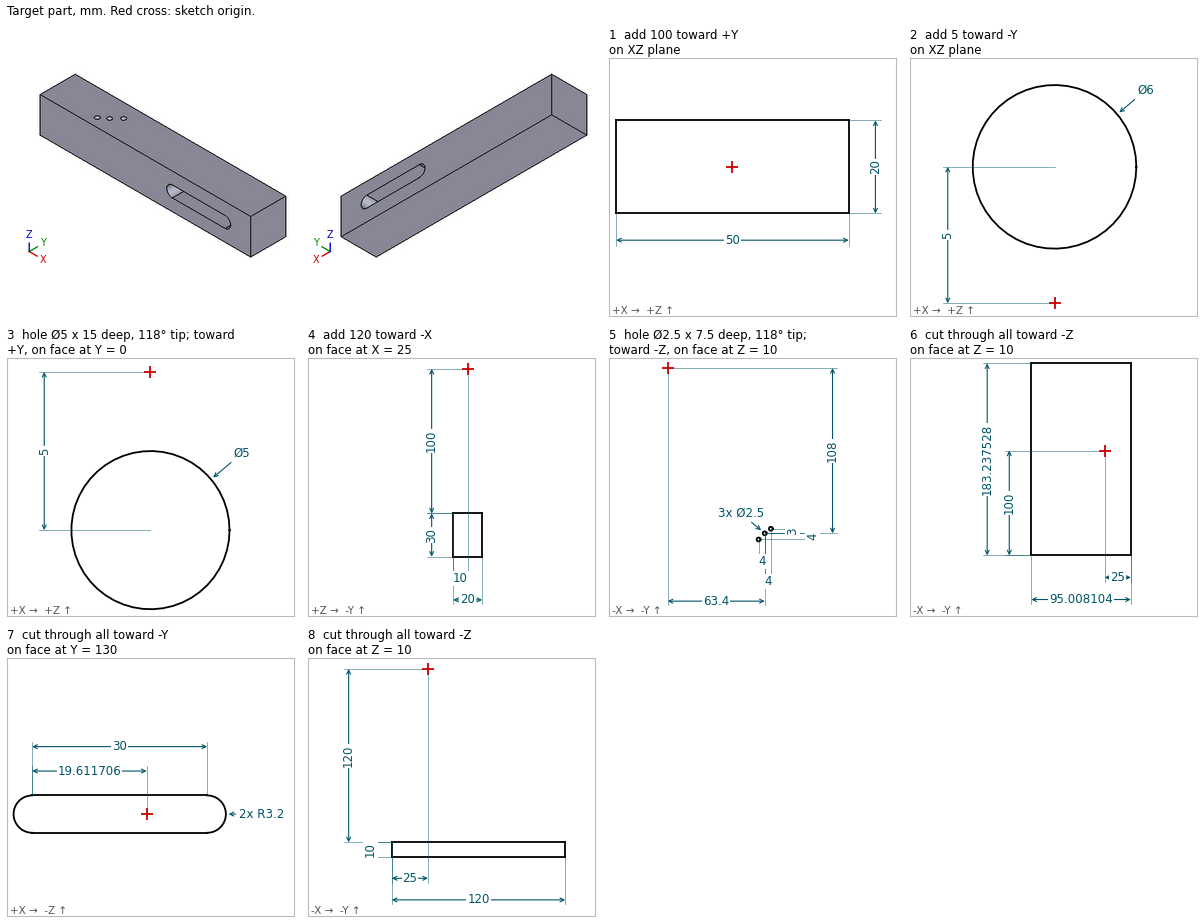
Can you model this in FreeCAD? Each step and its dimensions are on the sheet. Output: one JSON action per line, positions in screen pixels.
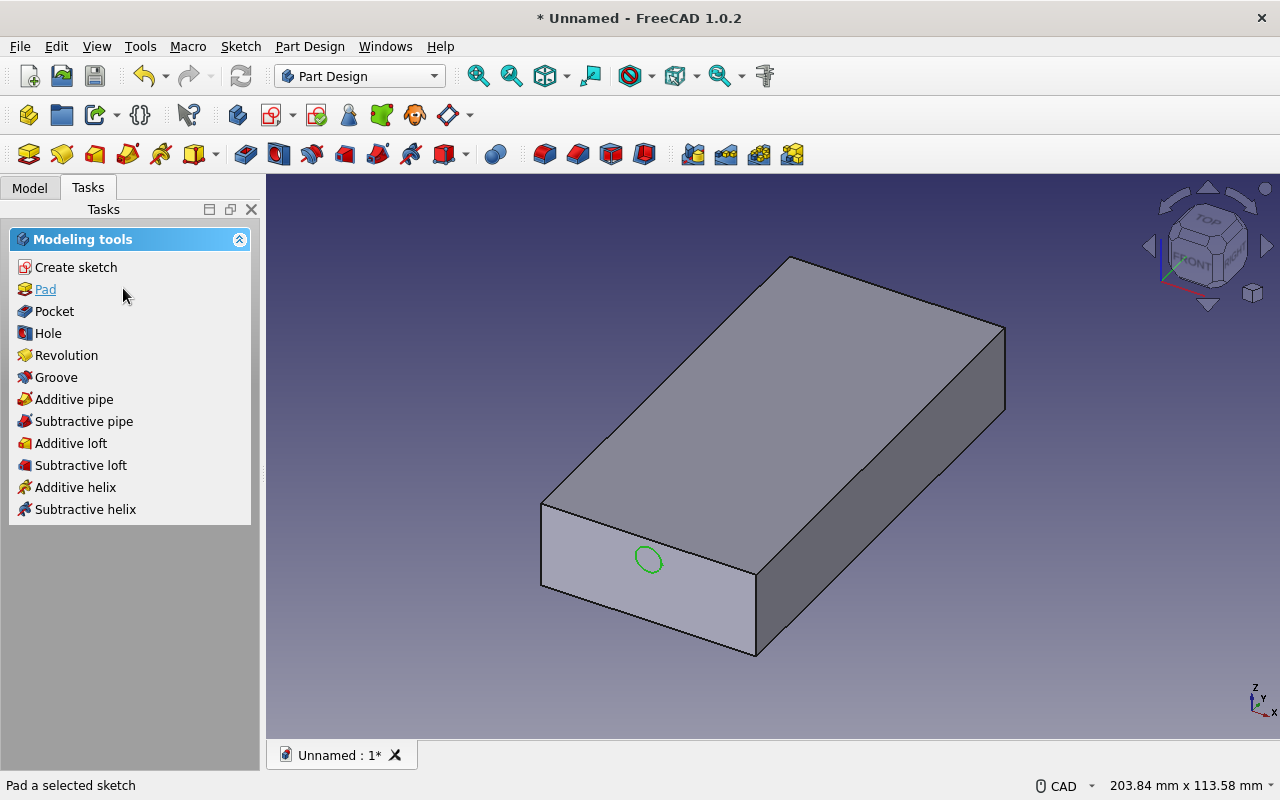
{"action": "left_click", "coordinate": [29, 154]}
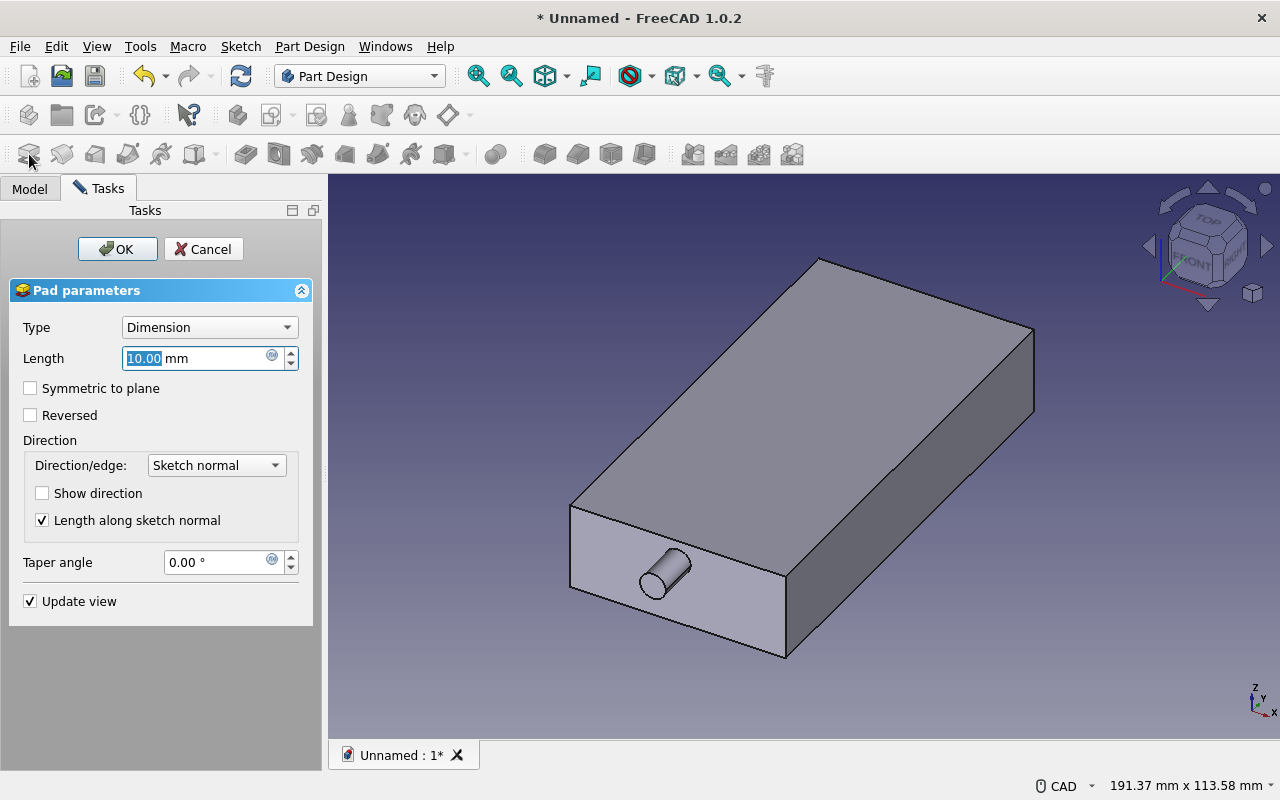
{"action": "type", "text": "5"}
{"action": "key", "text": "Tab"}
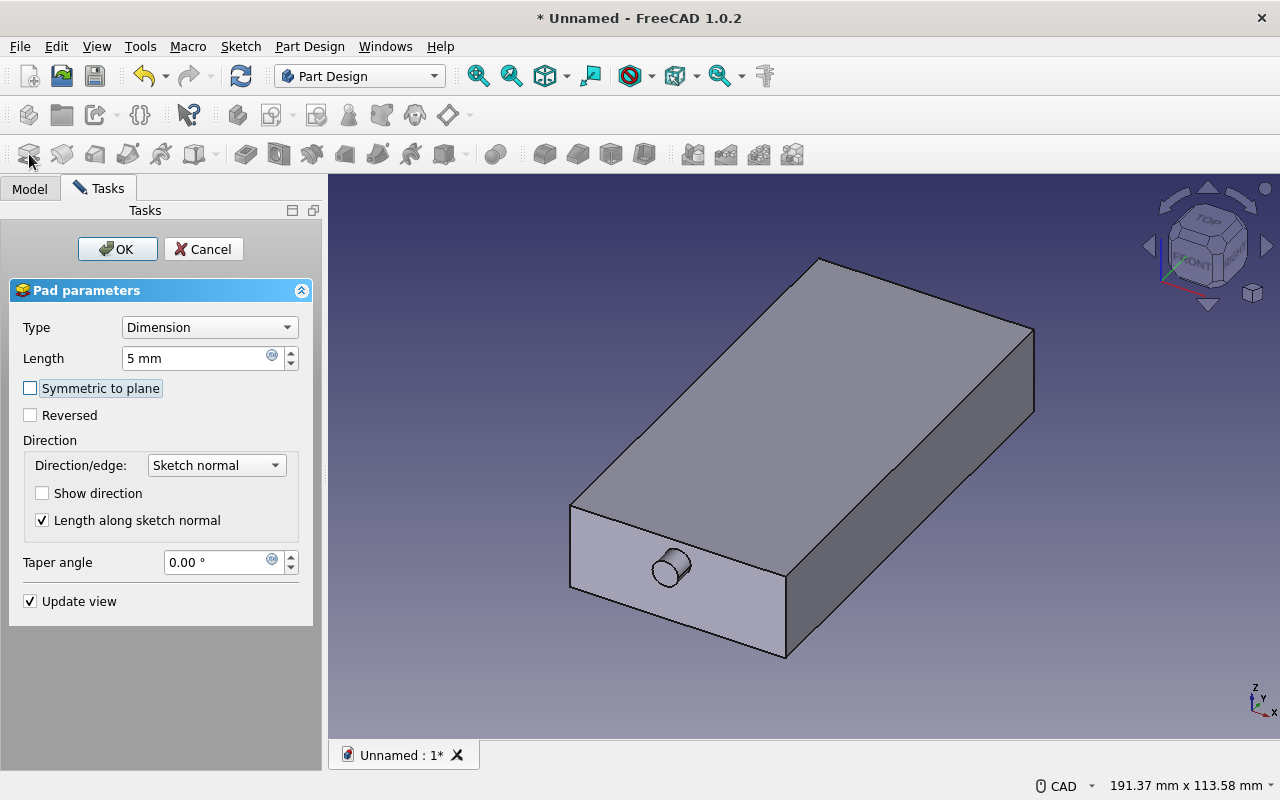
{"action": "left_click", "coordinate": [118, 249]}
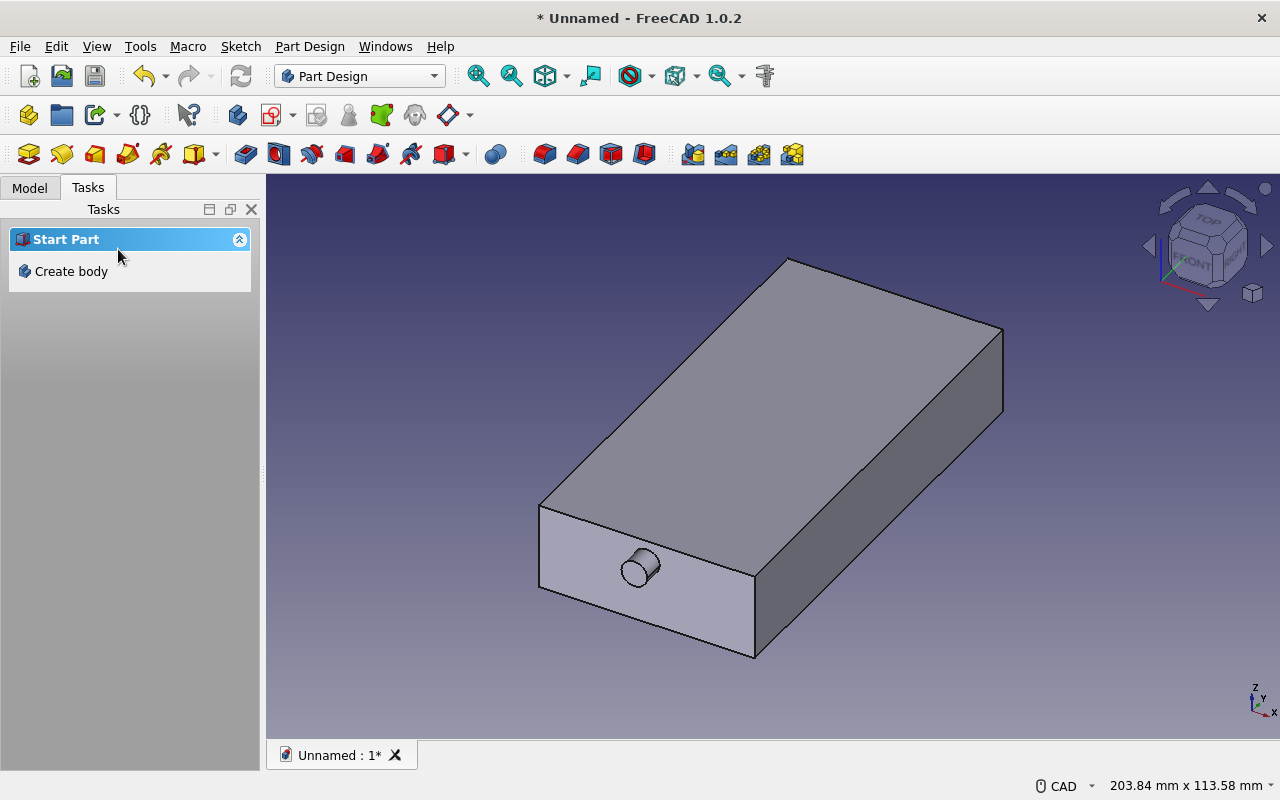
{"action": "left_click", "coordinate": [708, 601]}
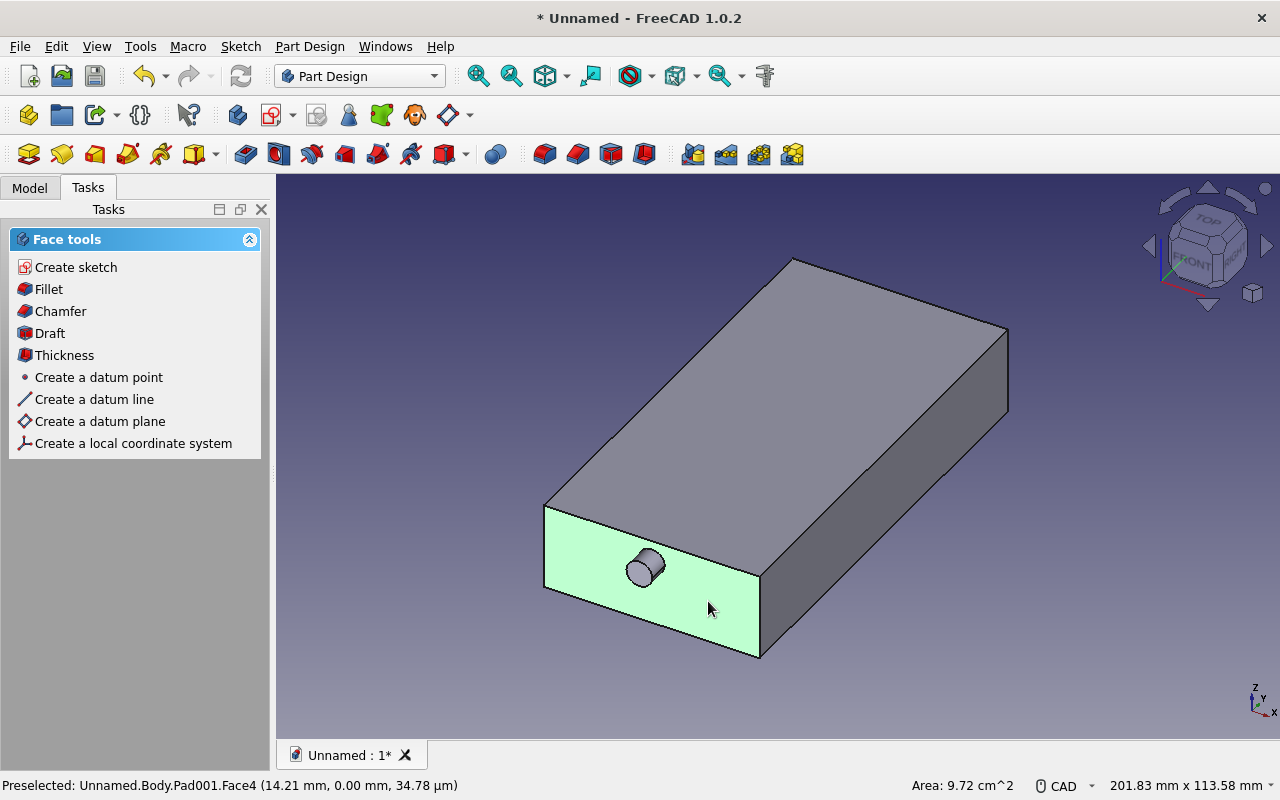
{"action": "left_click", "coordinate": [270, 116]}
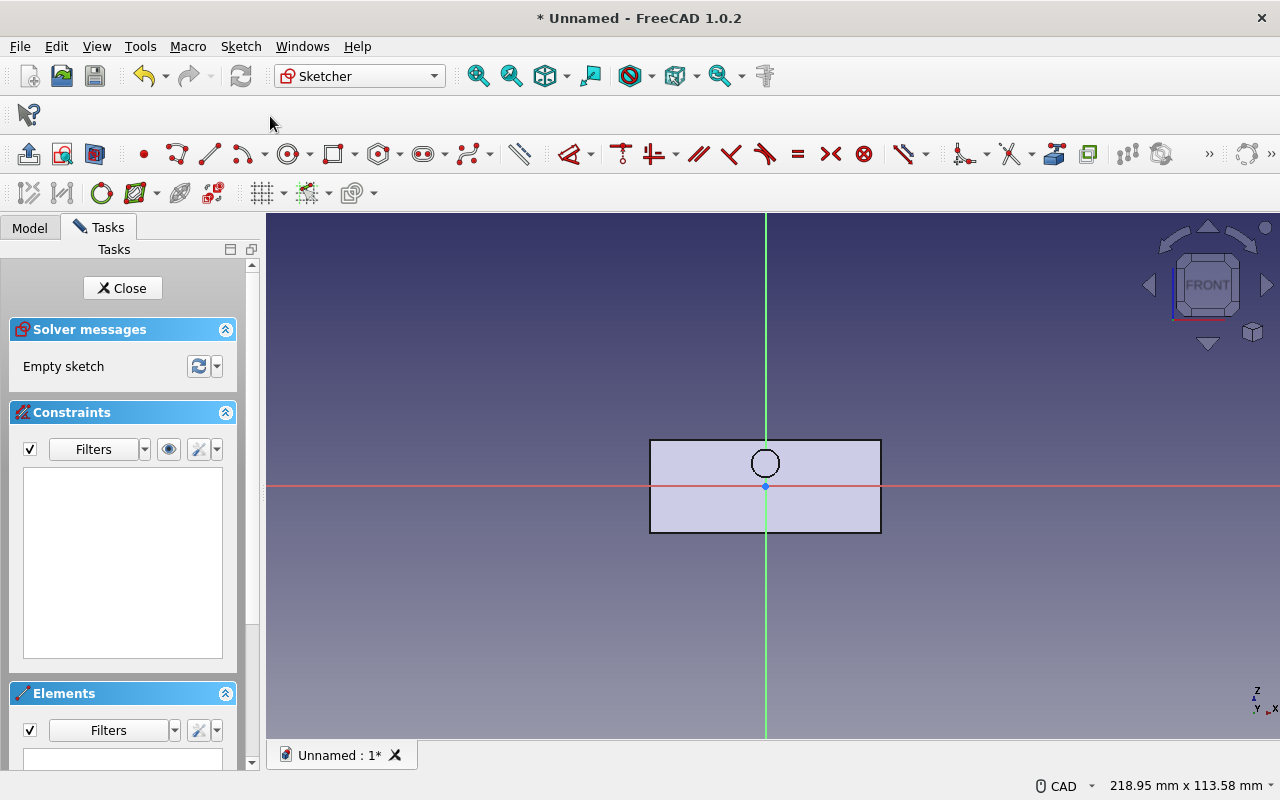
{"action": "scroll", "coordinate": [773, 507], "scroll_direction": "up", "scroll_amount": 11}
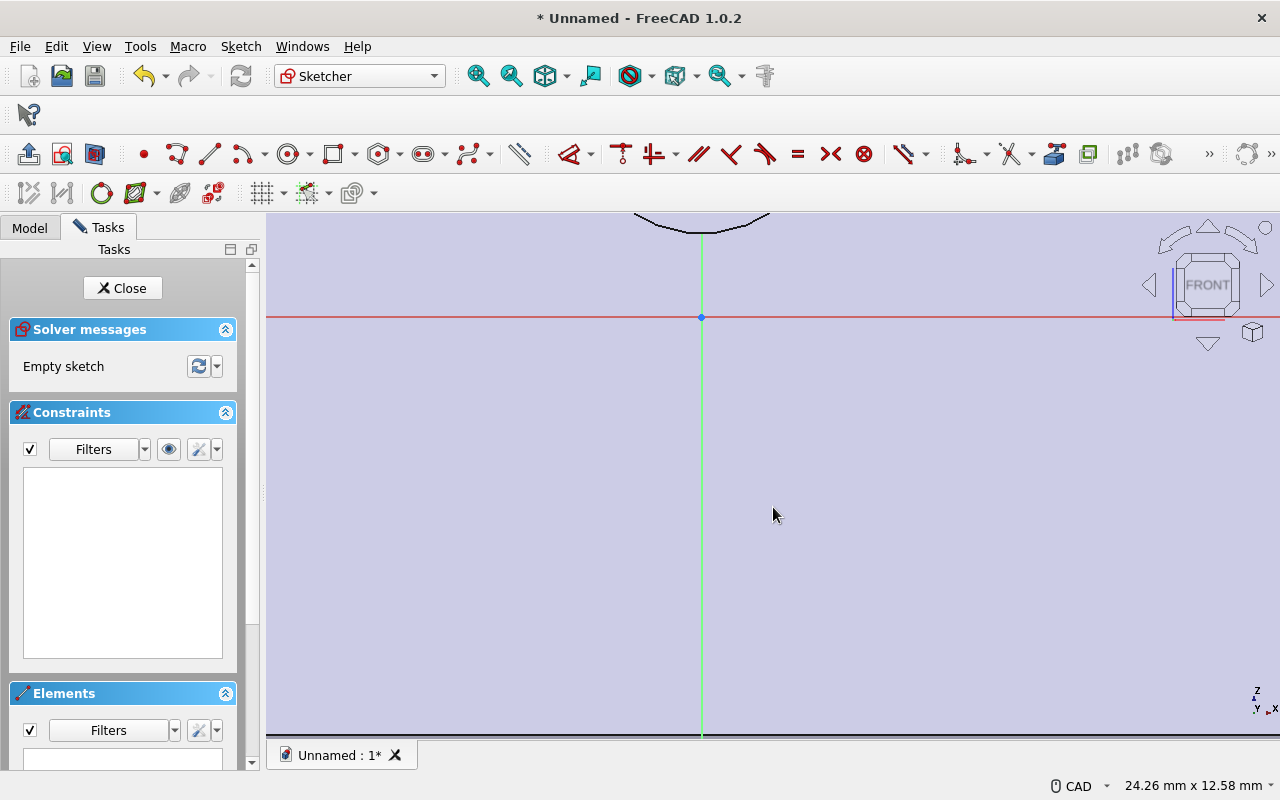
{"action": "left_click", "coordinate": [288, 154]}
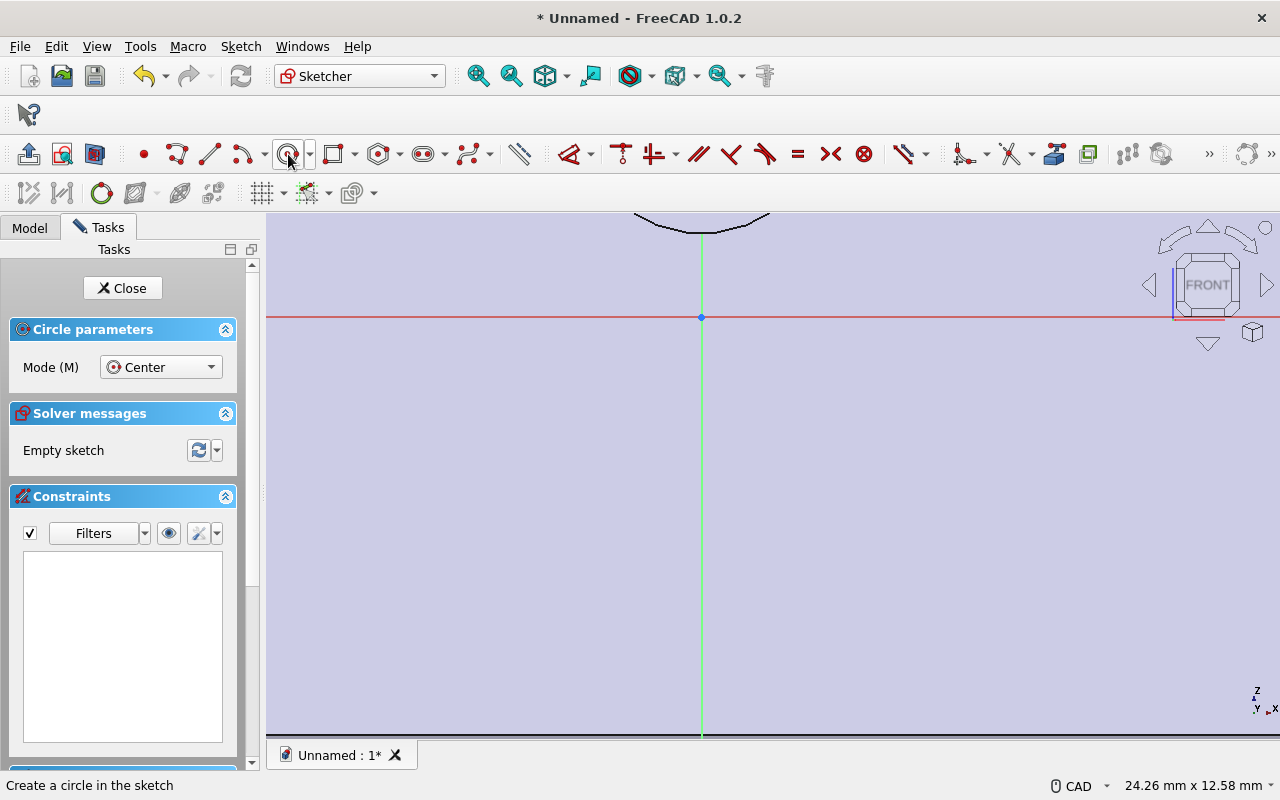
{"action": "left_click", "coordinate": [702, 526]}
{"action": "left_click", "coordinate": [775, 452]}
{"action": "key", "text": "Escape"}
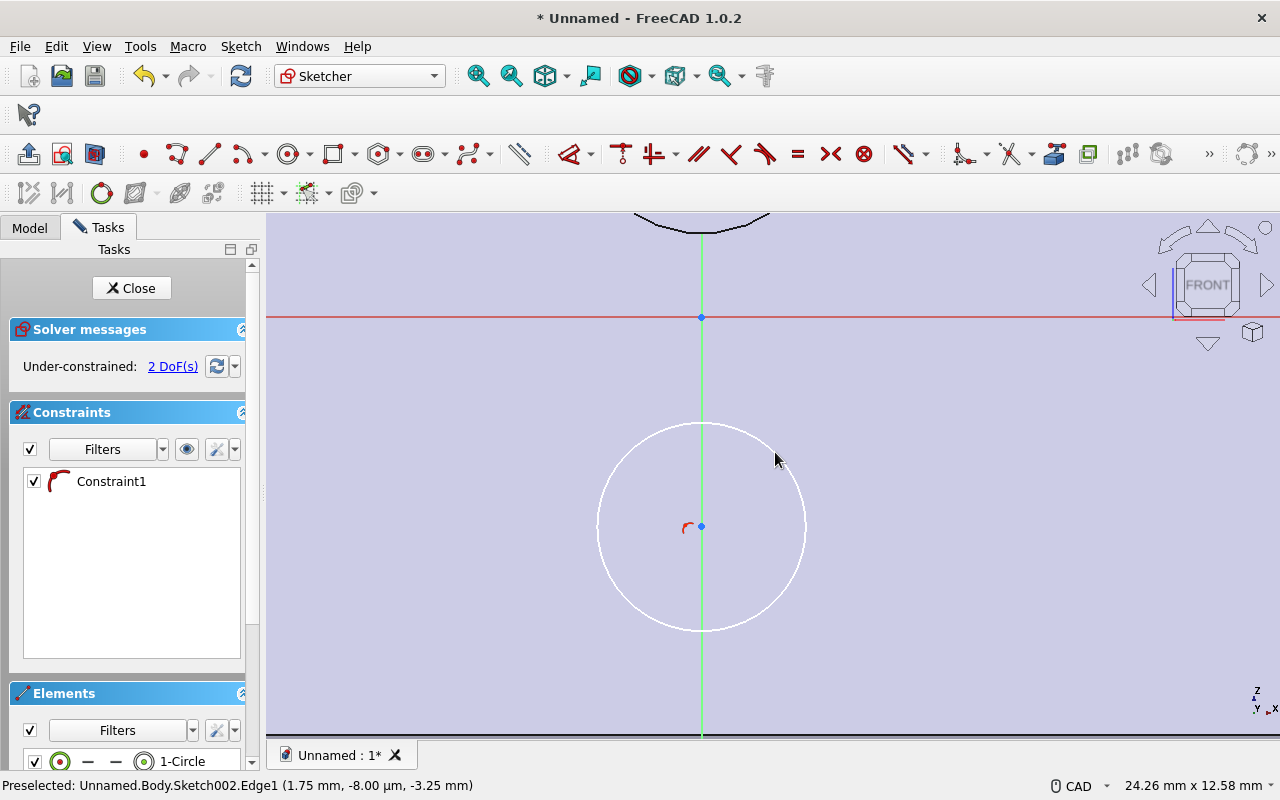
{"action": "key", "text": "d"}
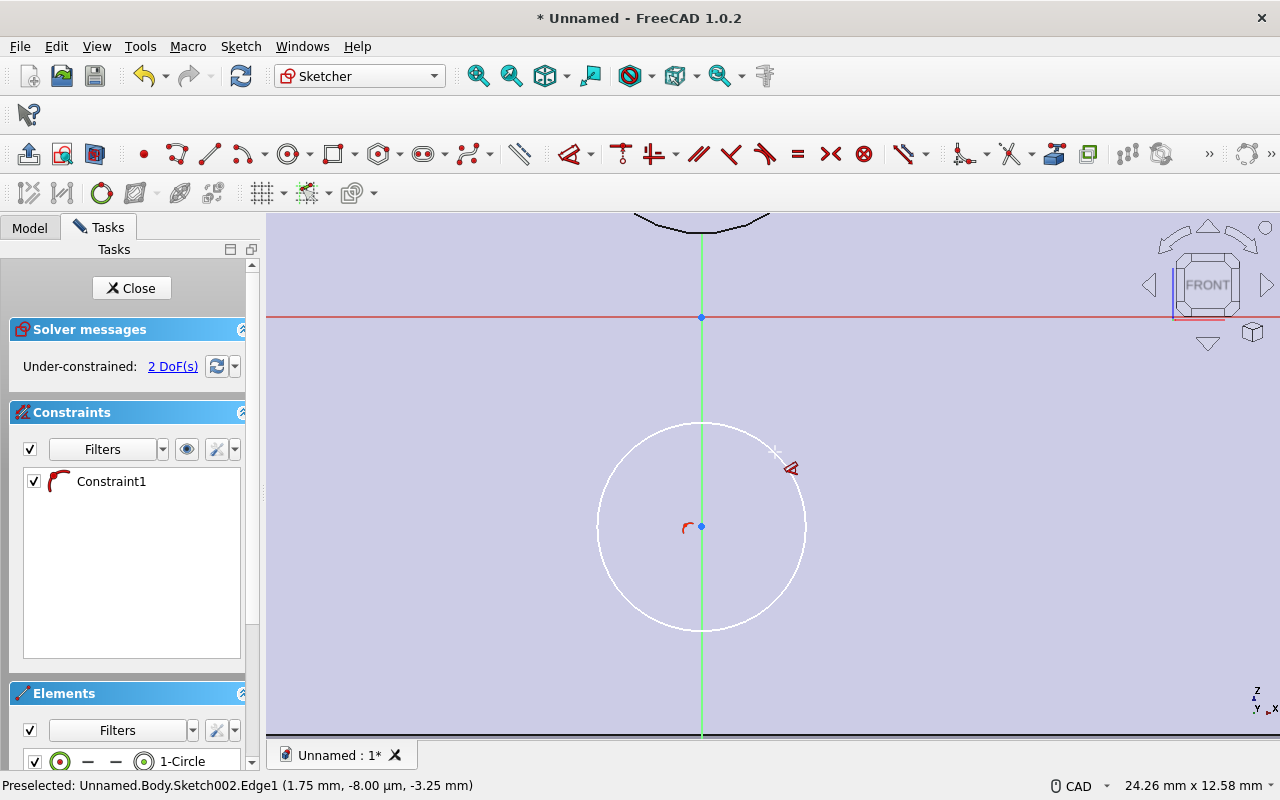
{"action": "left_click", "coordinate": [775, 453]}
{"action": "left_click", "coordinate": [798, 430]}